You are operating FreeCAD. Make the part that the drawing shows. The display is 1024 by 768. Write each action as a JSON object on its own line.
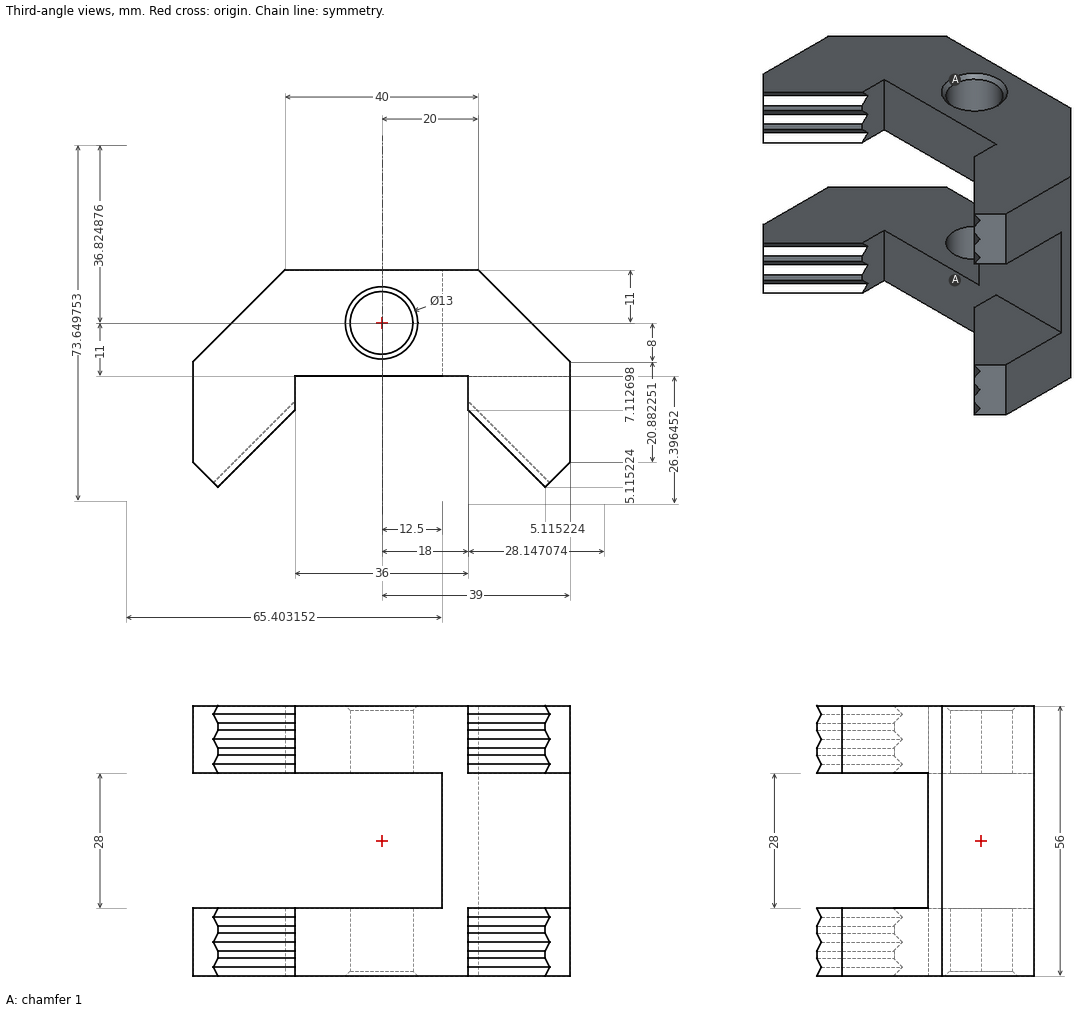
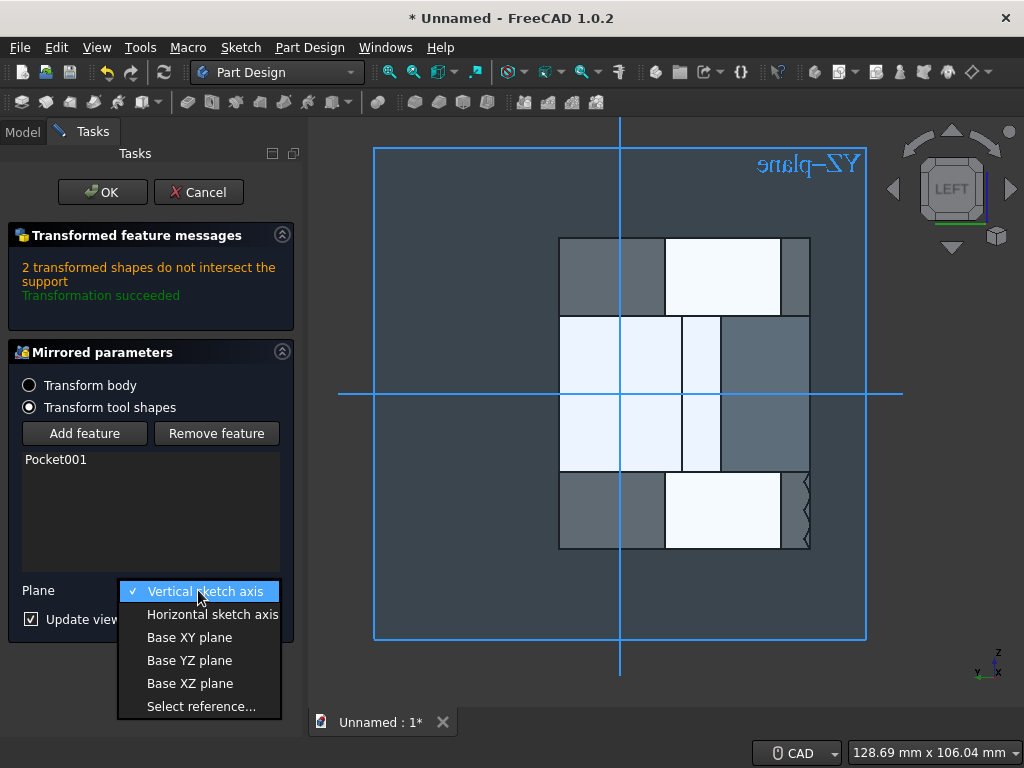
{"action": "left_click", "coordinate": [198, 638]}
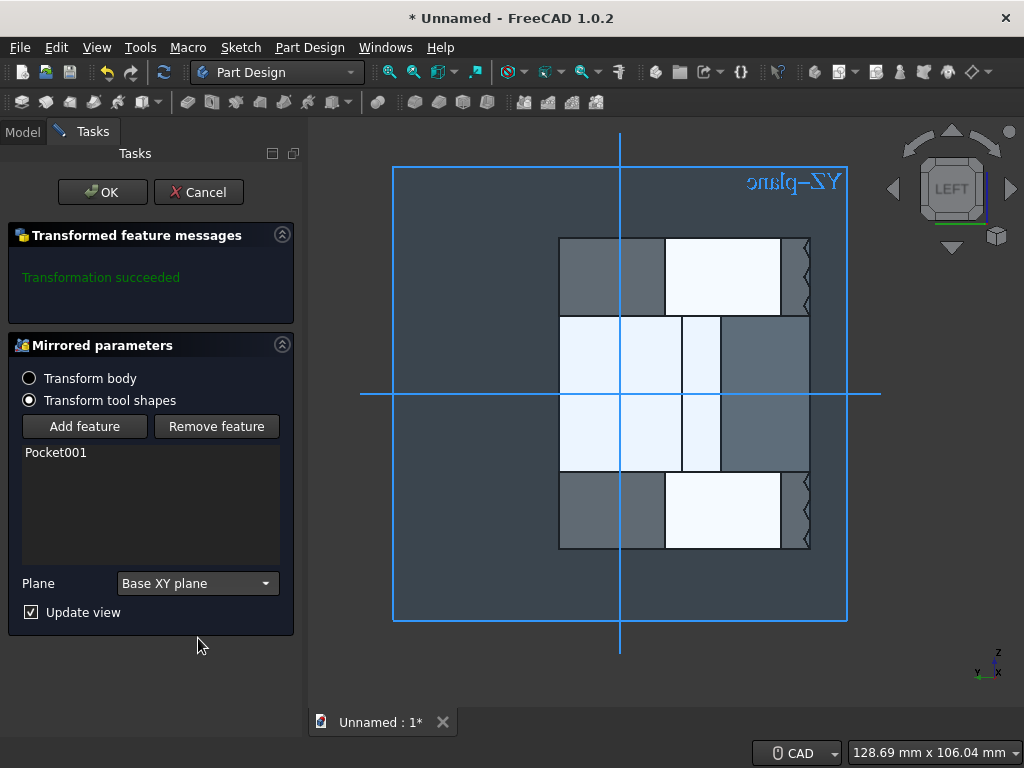
{"action": "left_click", "coordinate": [103, 192]}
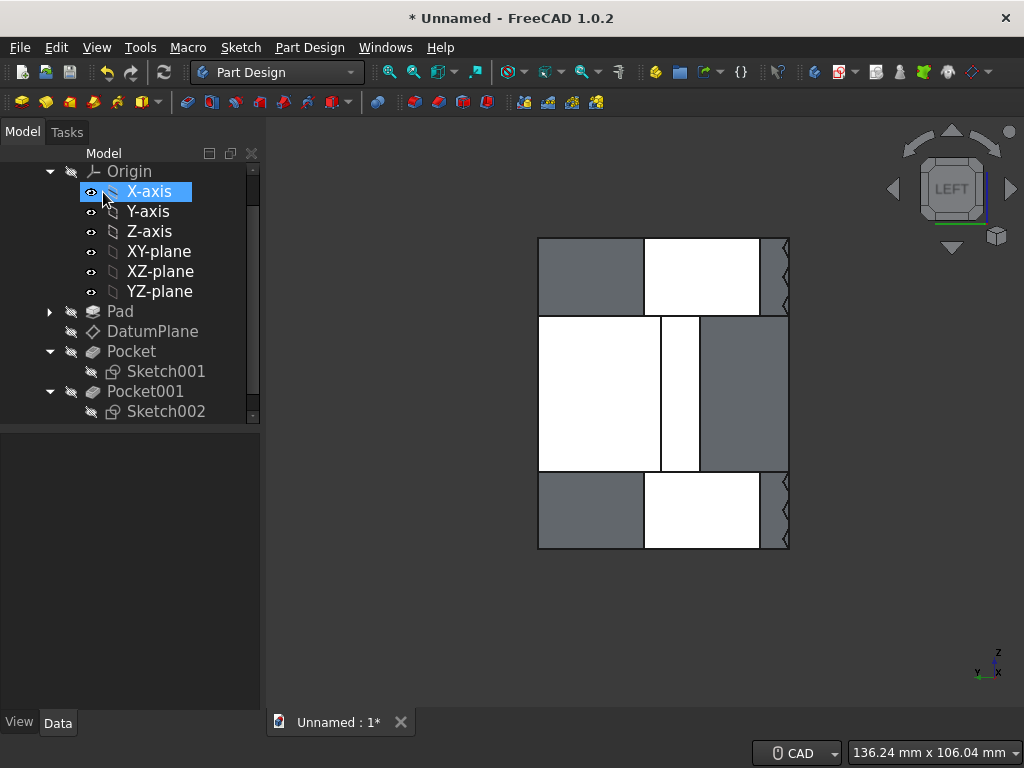
{"action": "left_click", "coordinate": [116, 392]}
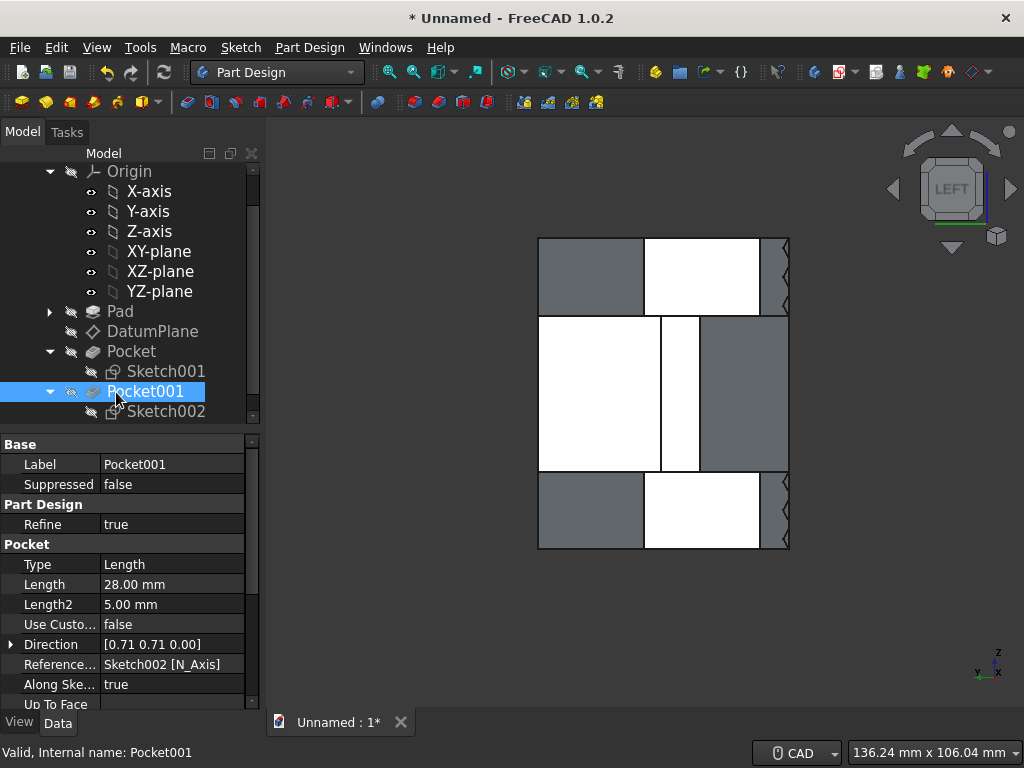
{"action": "left_click", "coordinate": [524, 102]}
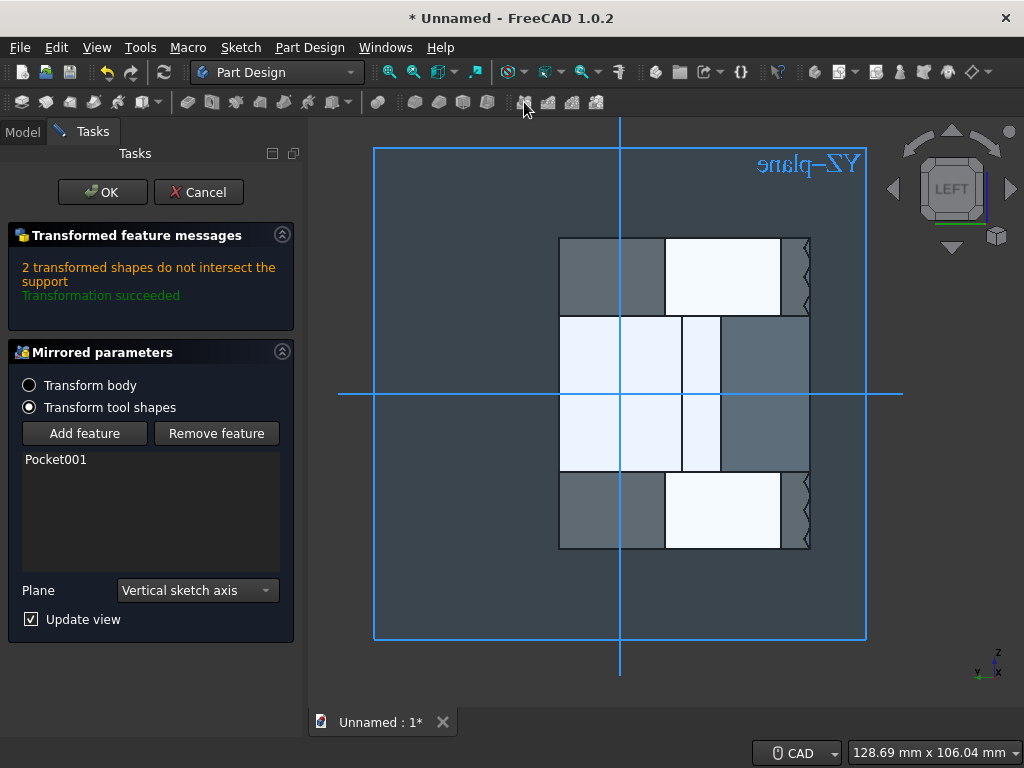
{"action": "left_click", "coordinate": [198, 590]}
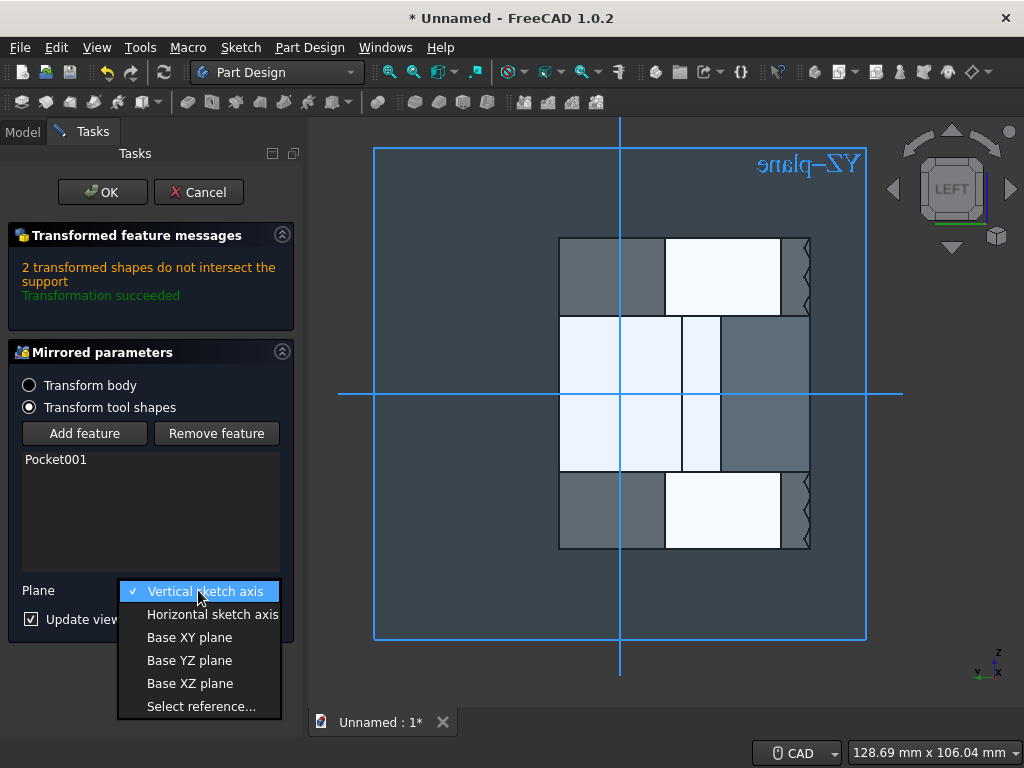
{"action": "left_click", "coordinate": [198, 660]}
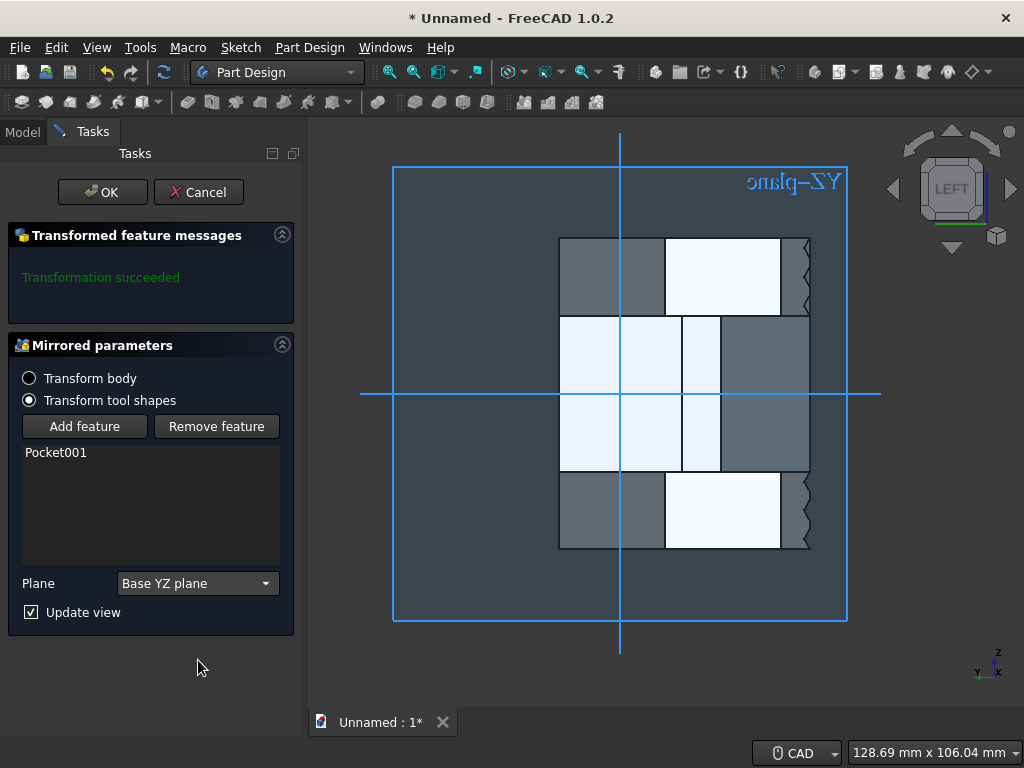
{"action": "left_click", "coordinate": [103, 192]}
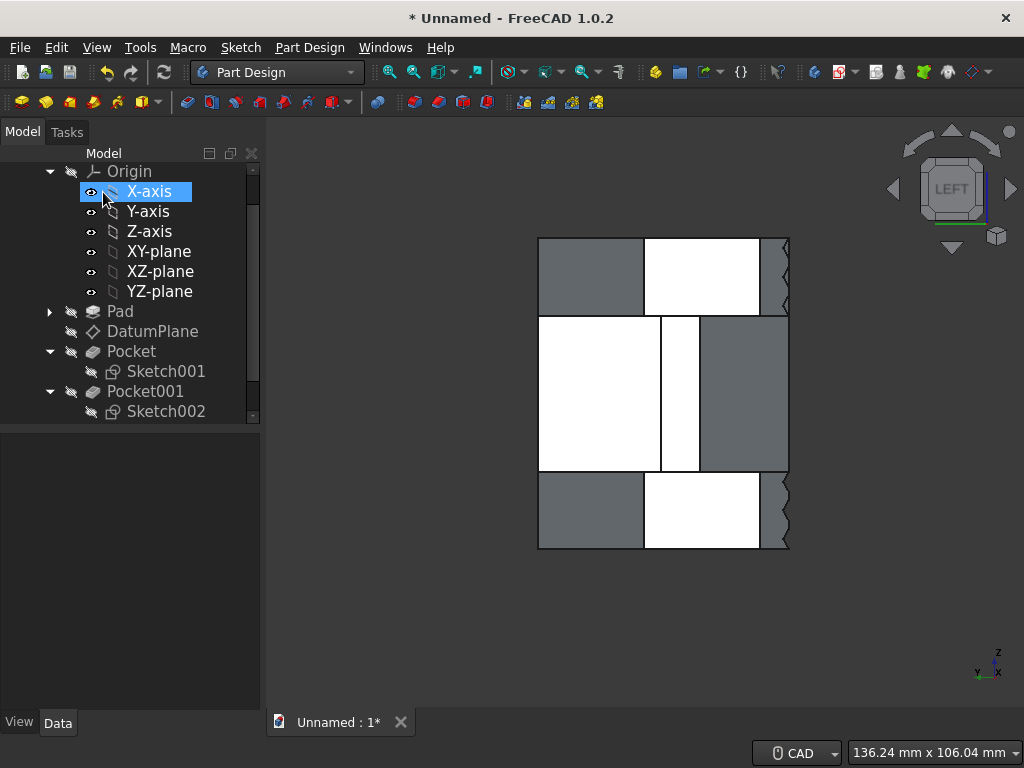
{"action": "key", "text": "0"}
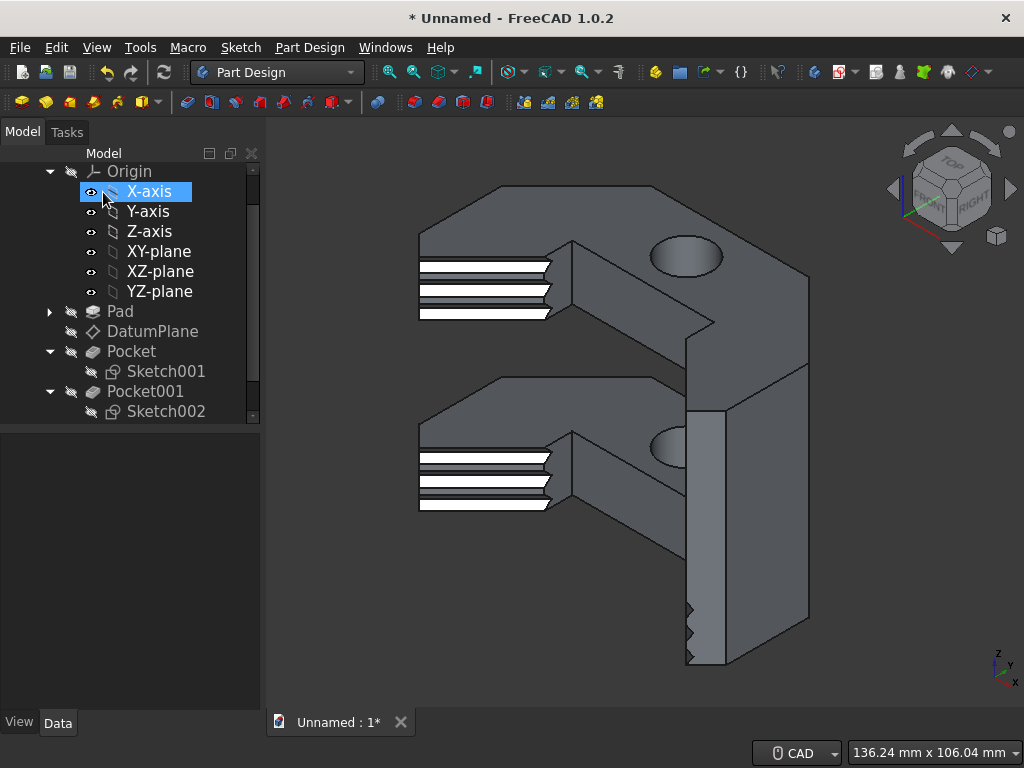
{"action": "left_click", "coordinate": [706, 428]}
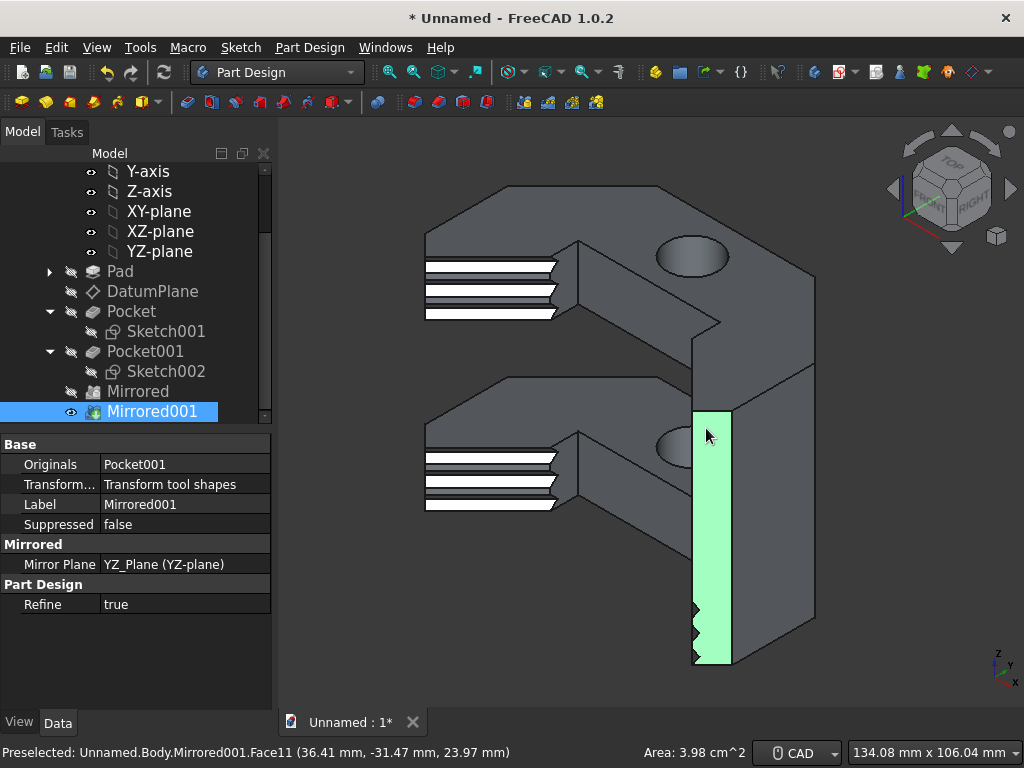
{"action": "left_click", "coordinate": [840, 72]}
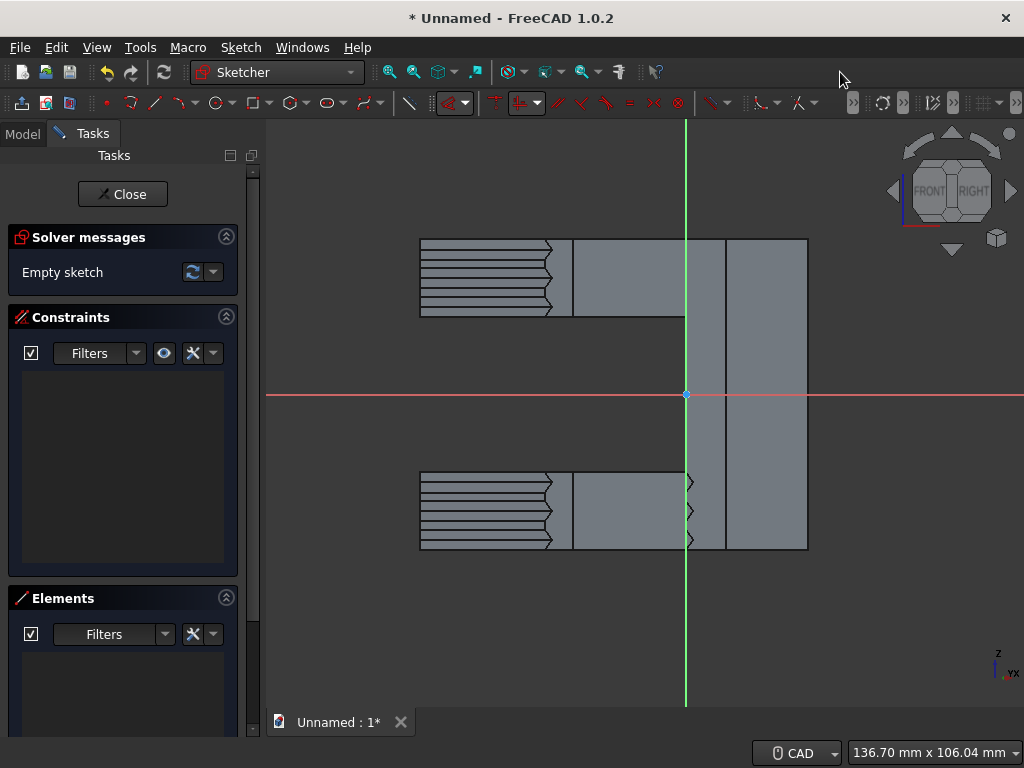
{"action": "scroll", "coordinate": [782, 239], "scroll_direction": "up", "scroll_amount": 4}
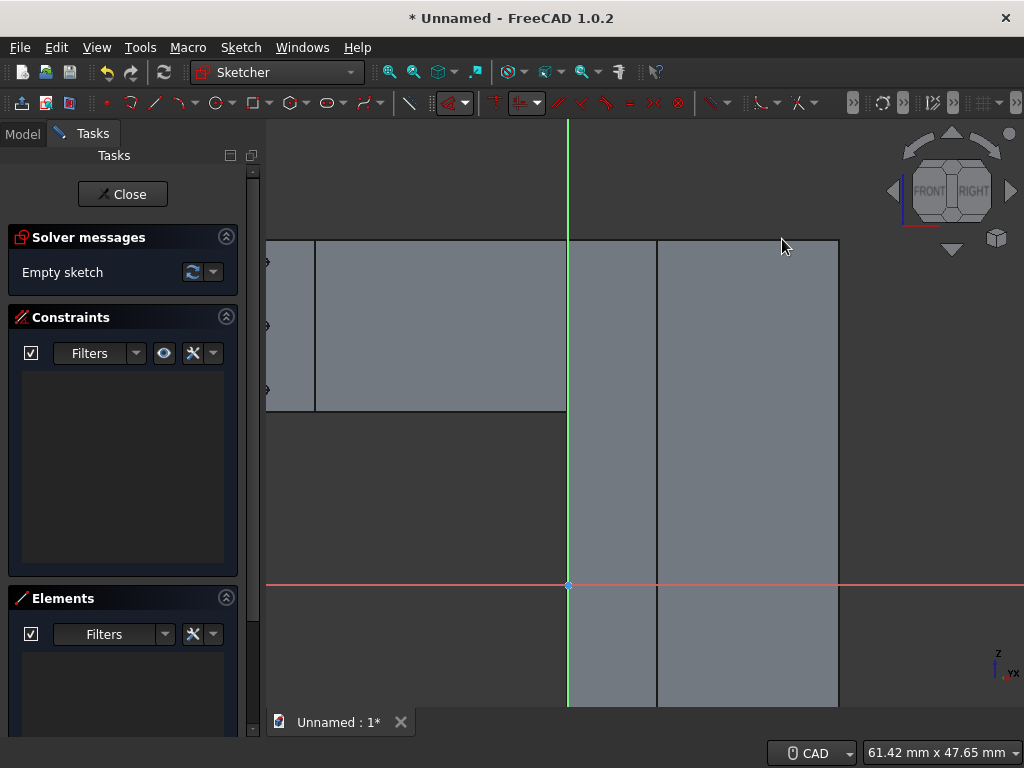
{"action": "left_click", "coordinate": [132, 104]}